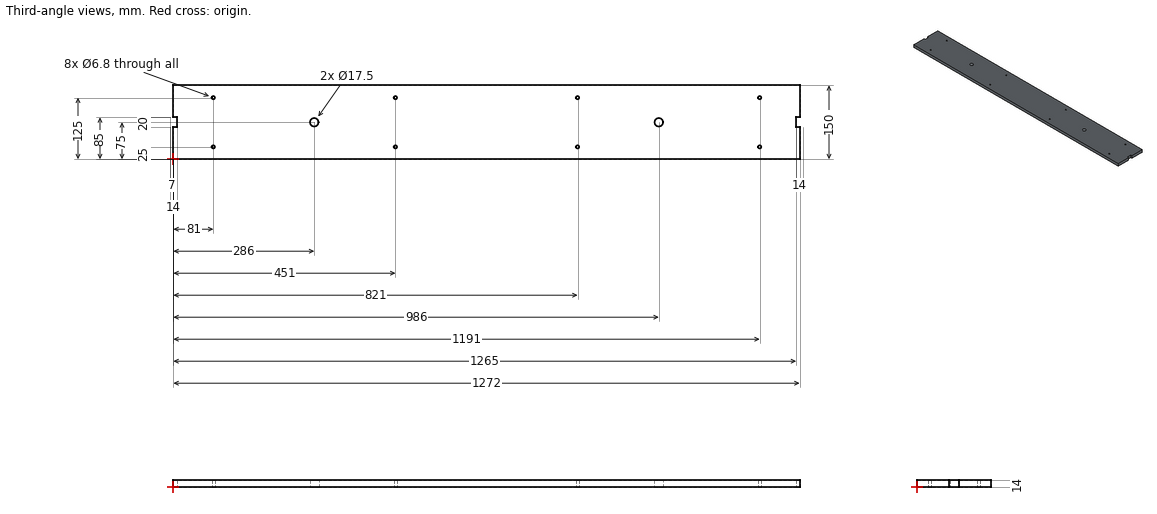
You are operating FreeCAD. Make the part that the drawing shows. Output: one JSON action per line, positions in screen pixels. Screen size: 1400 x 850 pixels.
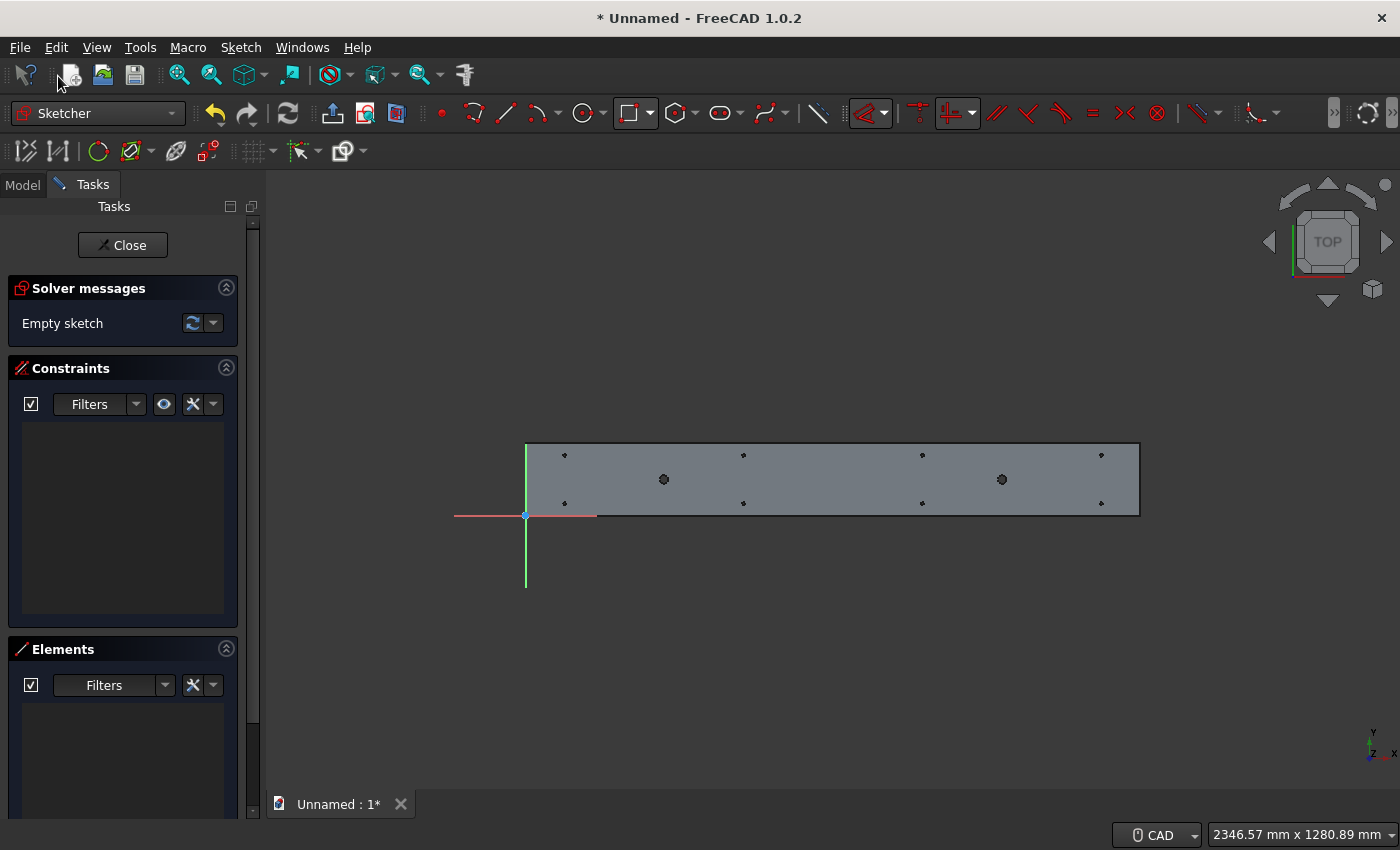
{"action": "left_click", "coordinate": [630, 114]}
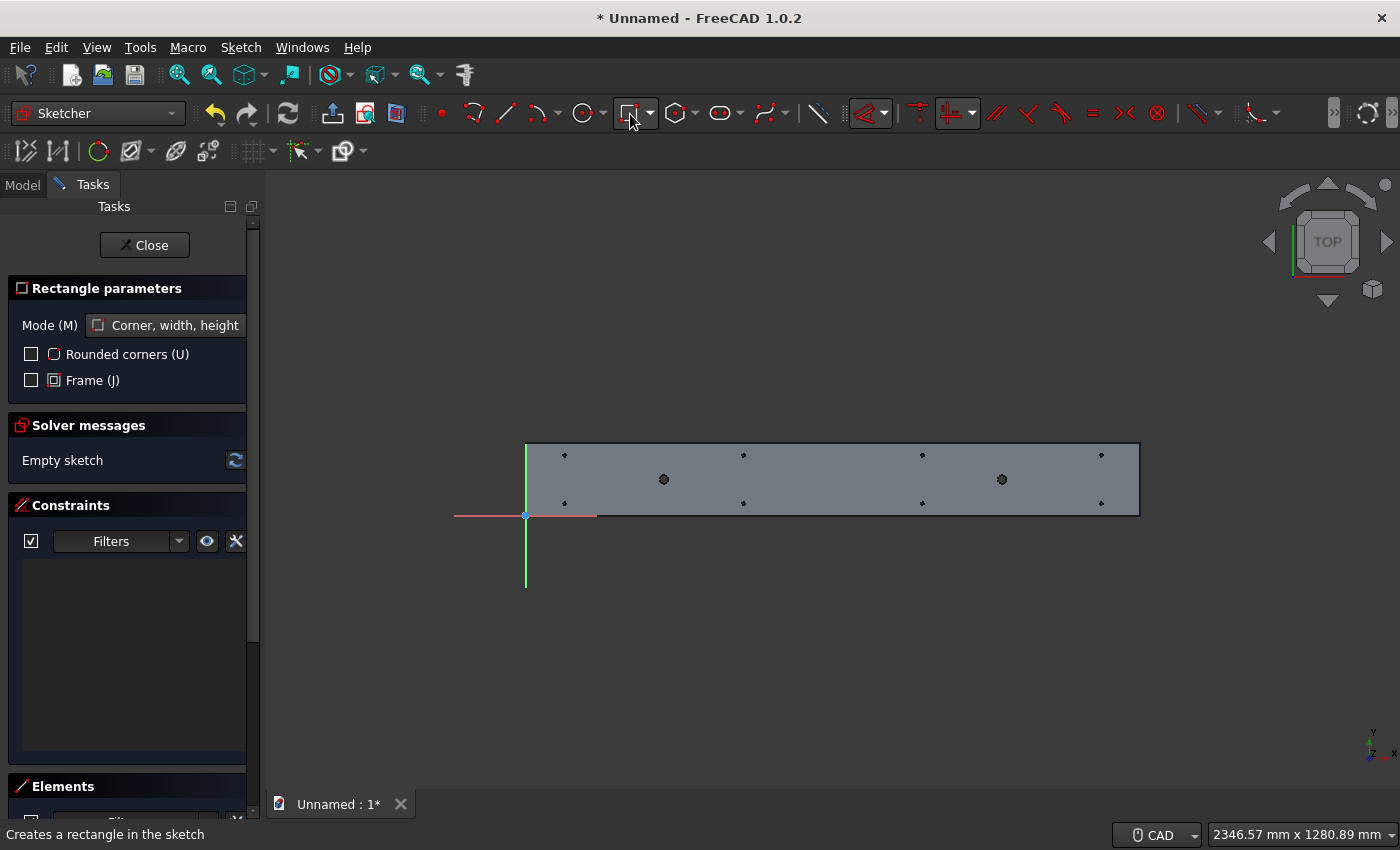
{"action": "scroll", "coordinate": [522, 475], "scroll_direction": "up", "scroll_amount": 8}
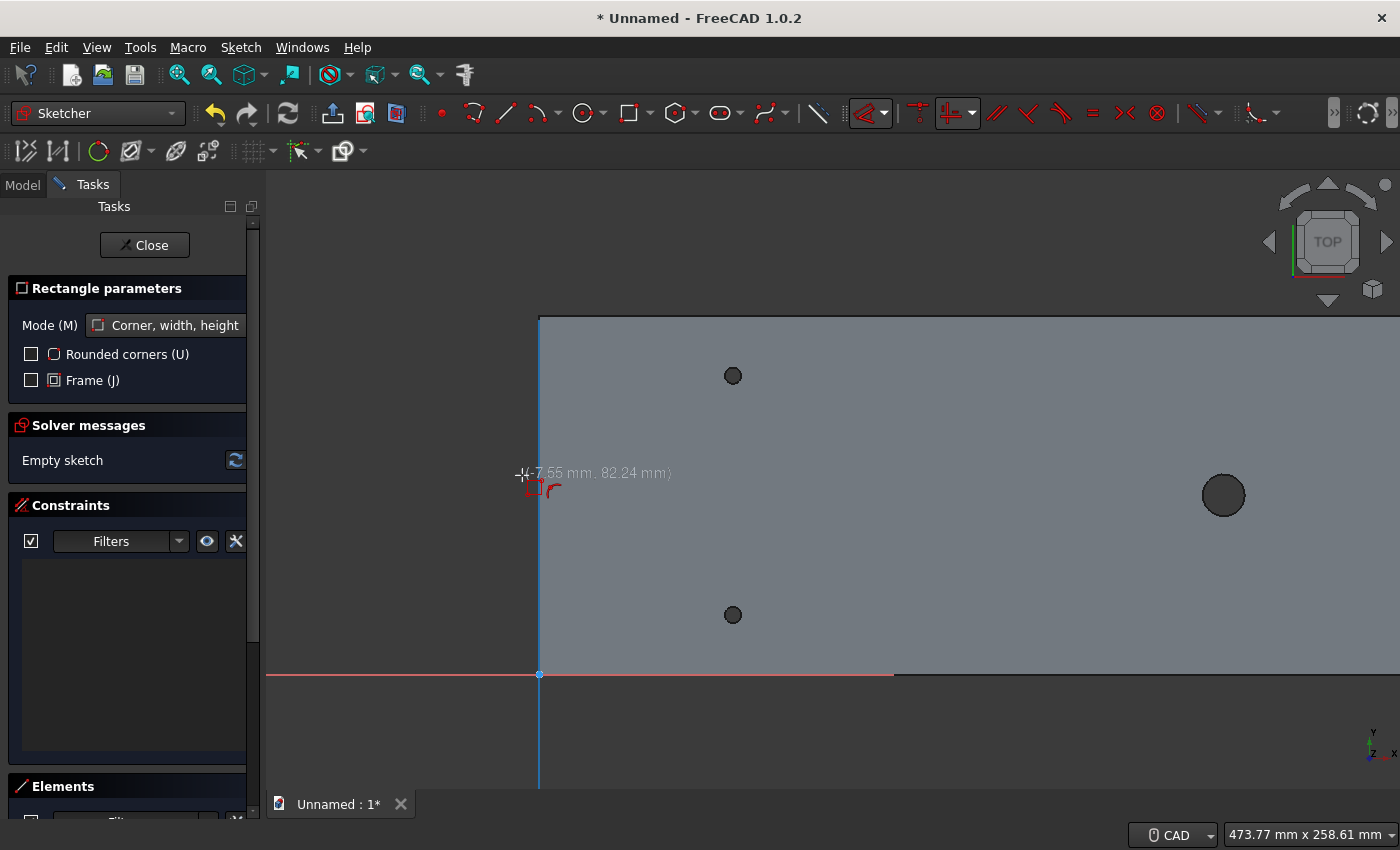
{"action": "left_click", "coordinate": [522, 471]}
{"action": "left_click", "coordinate": [556, 519]}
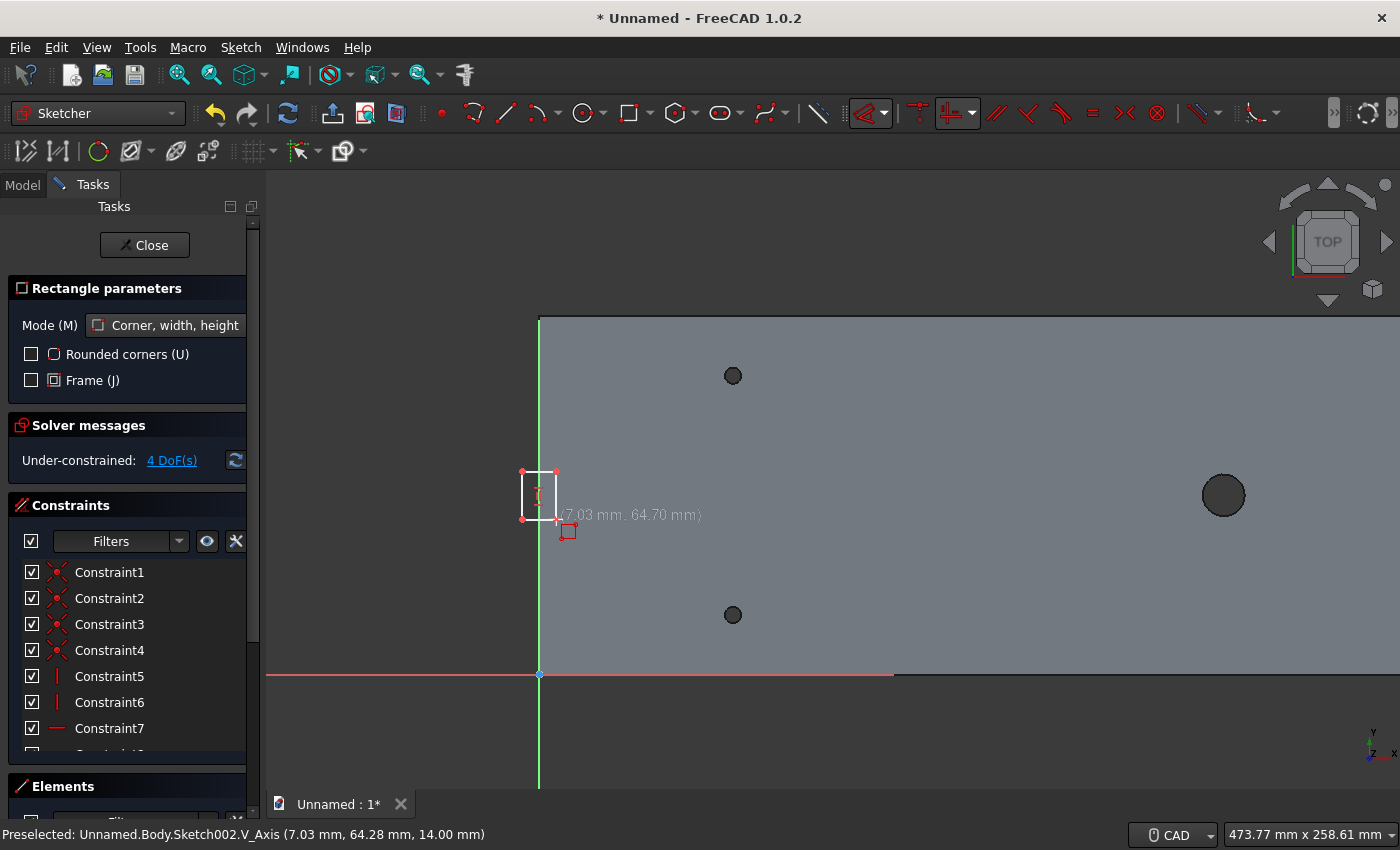
{"action": "scroll", "coordinate": [436, 456], "scroll_direction": "down", "scroll_amount": 8}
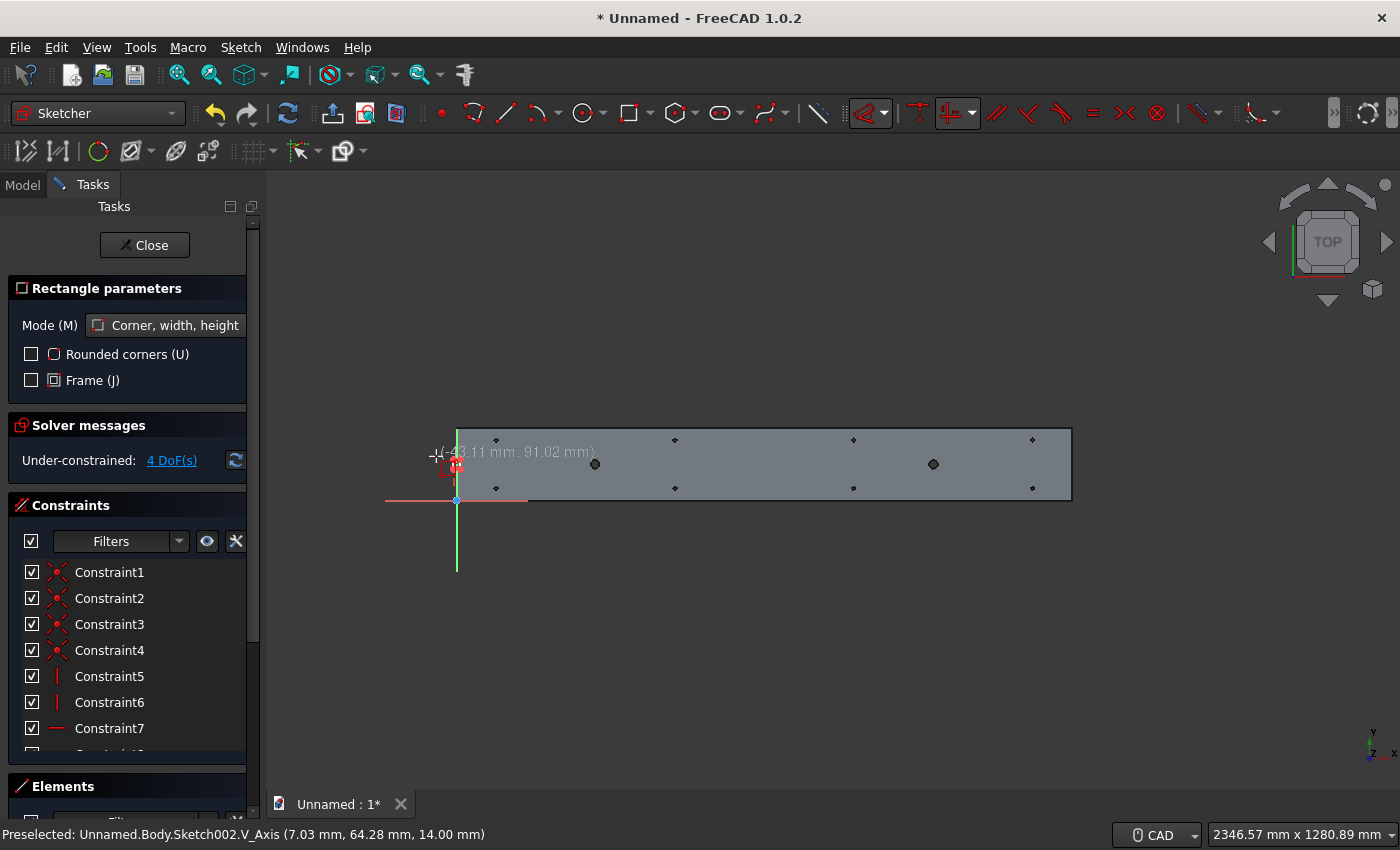
{"action": "scroll", "coordinate": [1068, 459], "scroll_direction": "up", "scroll_amount": 5}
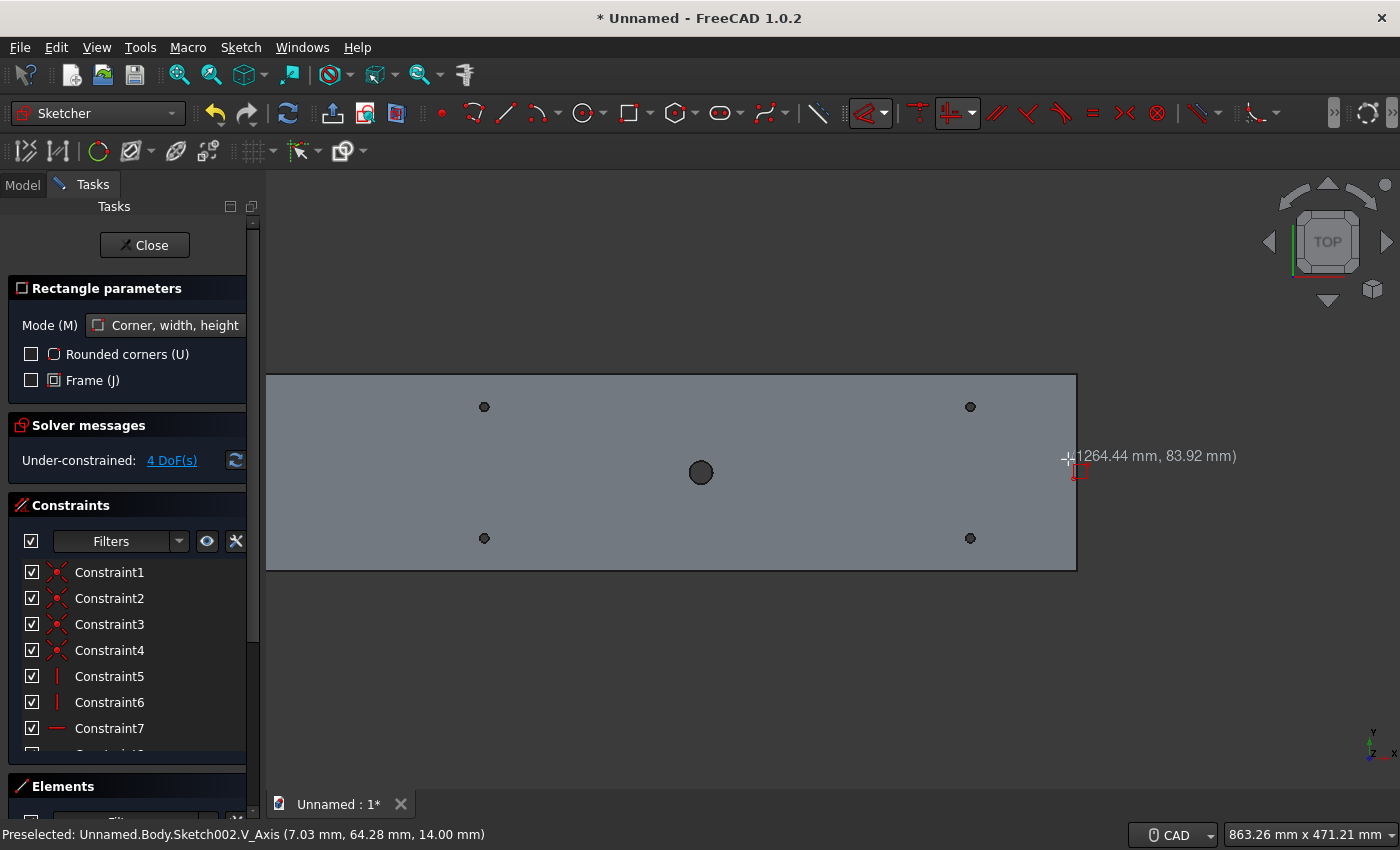
{"action": "left_click", "coordinate": [1068, 459]}
{"action": "left_click", "coordinate": [1086, 486]}
{"action": "key", "text": "Escape"}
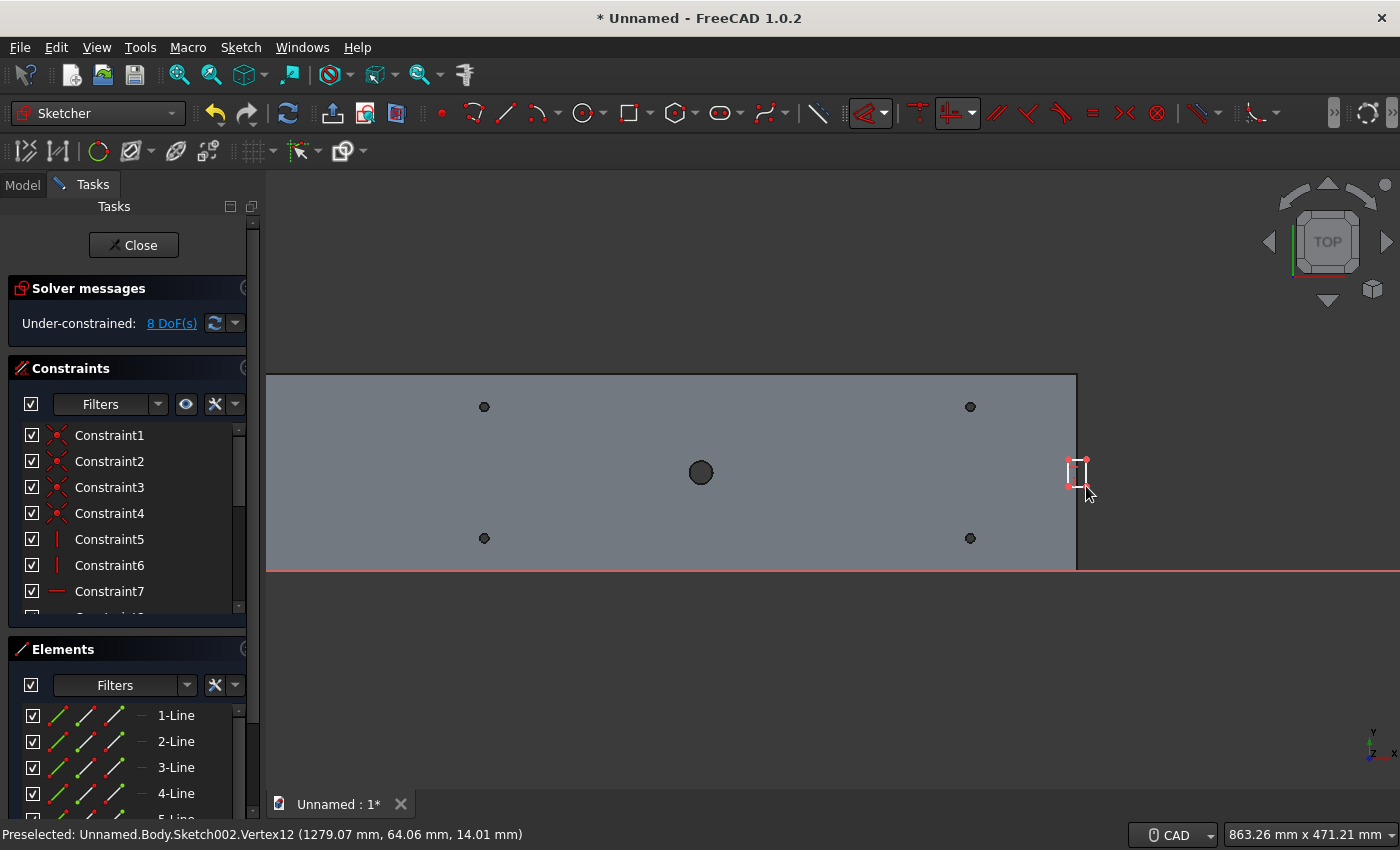
{"action": "scroll", "coordinate": [1069, 459], "scroll_direction": "down", "scroll_amount": 5}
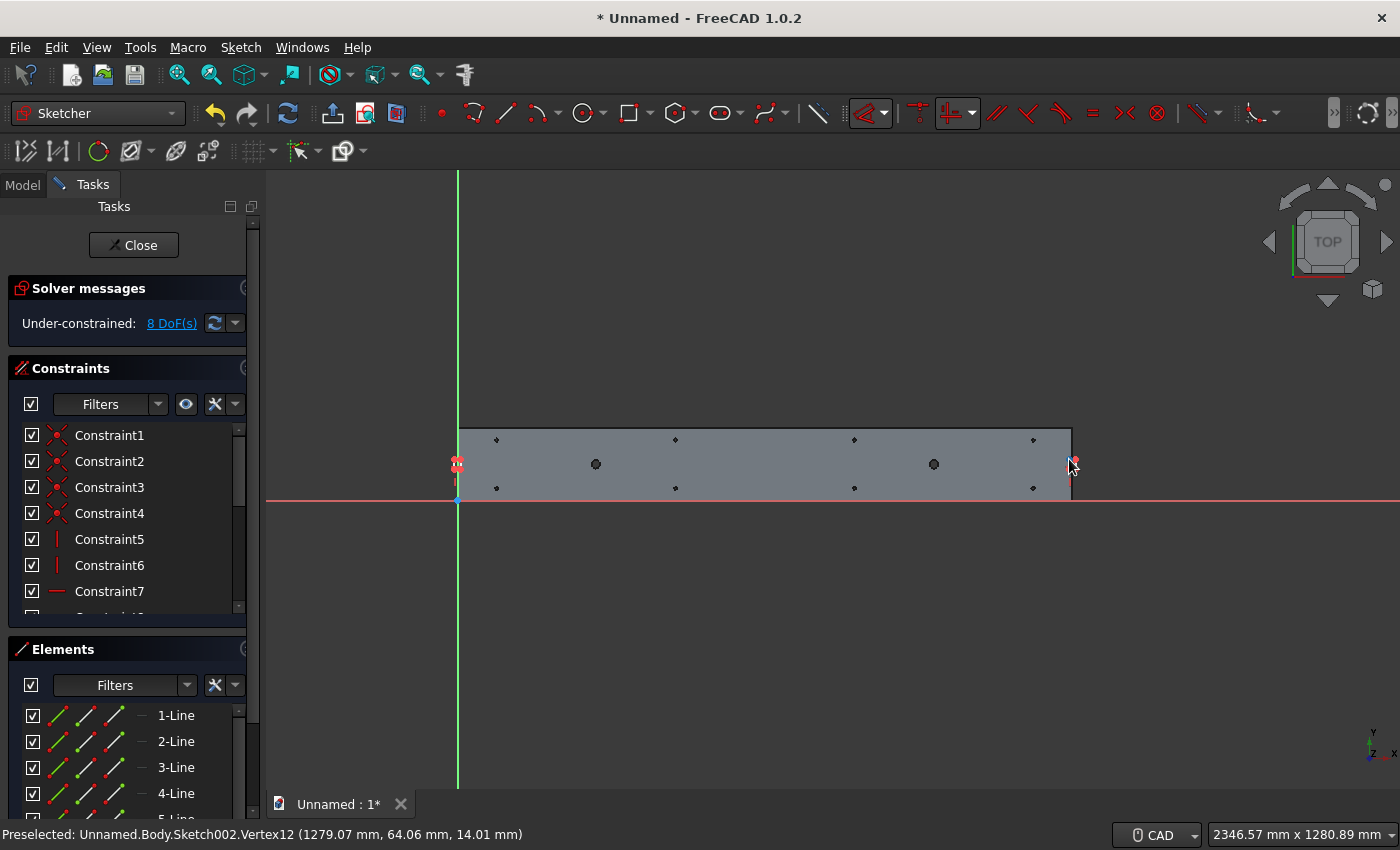
{"action": "scroll", "coordinate": [454, 463], "scroll_direction": "up", "scroll_amount": 8}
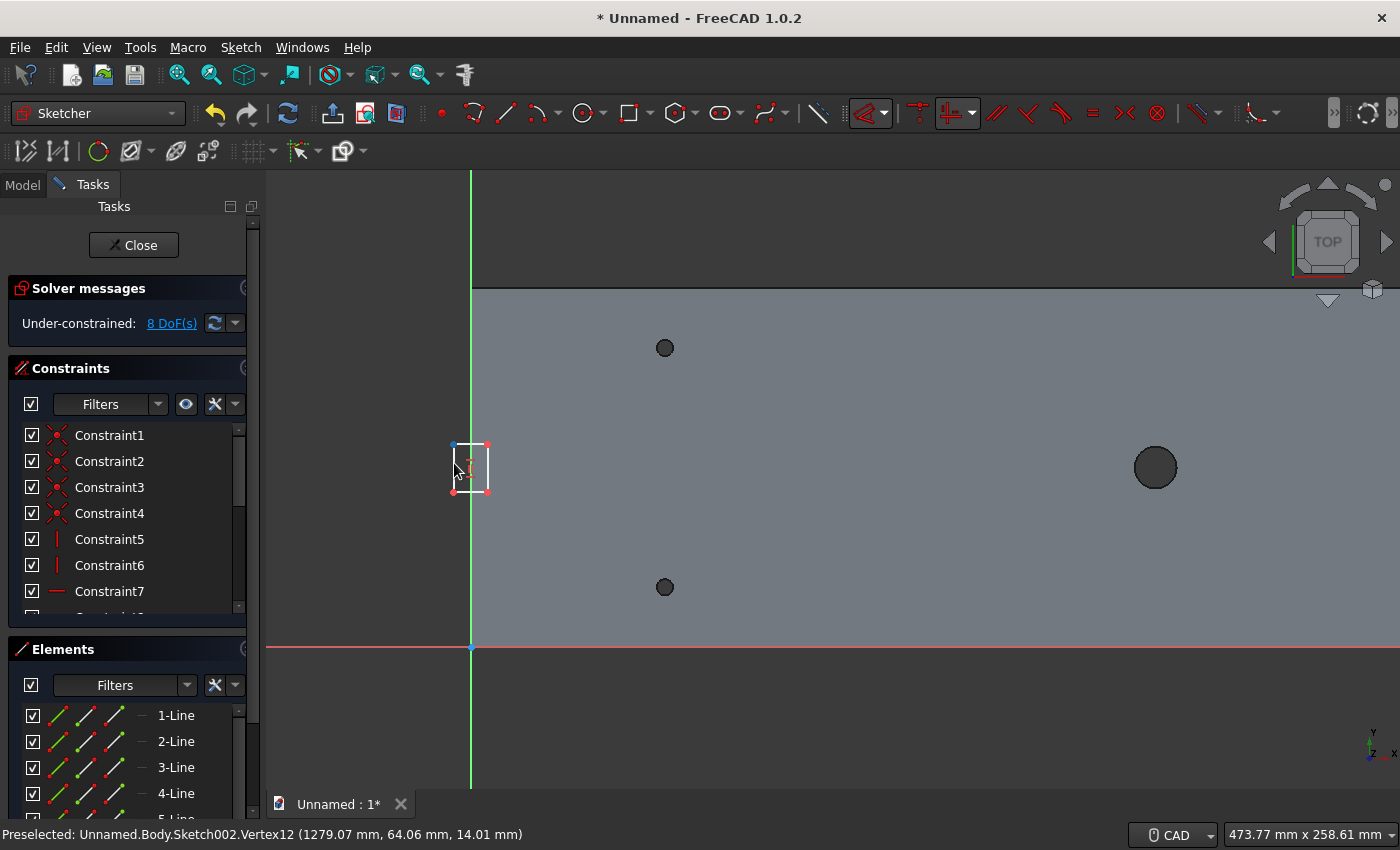
{"action": "left_click", "coordinate": [454, 463]}